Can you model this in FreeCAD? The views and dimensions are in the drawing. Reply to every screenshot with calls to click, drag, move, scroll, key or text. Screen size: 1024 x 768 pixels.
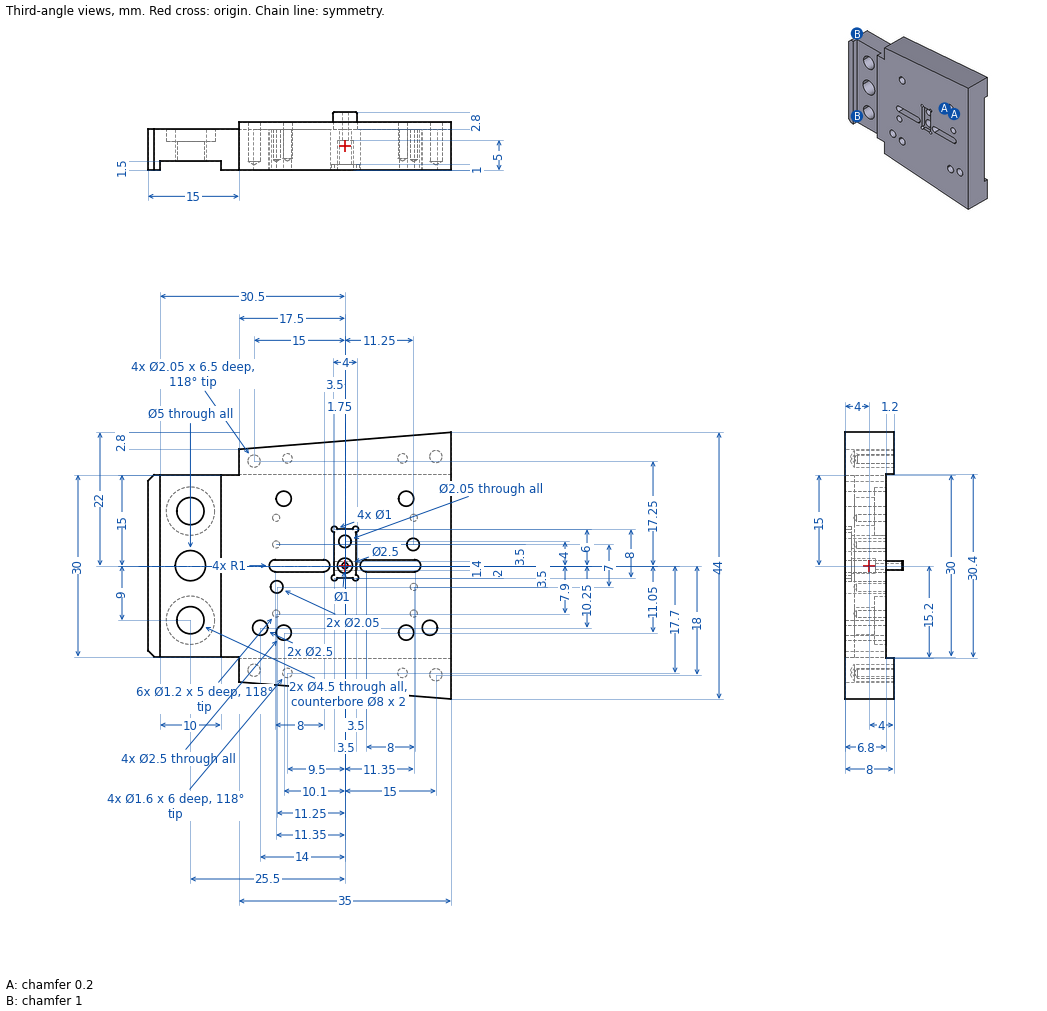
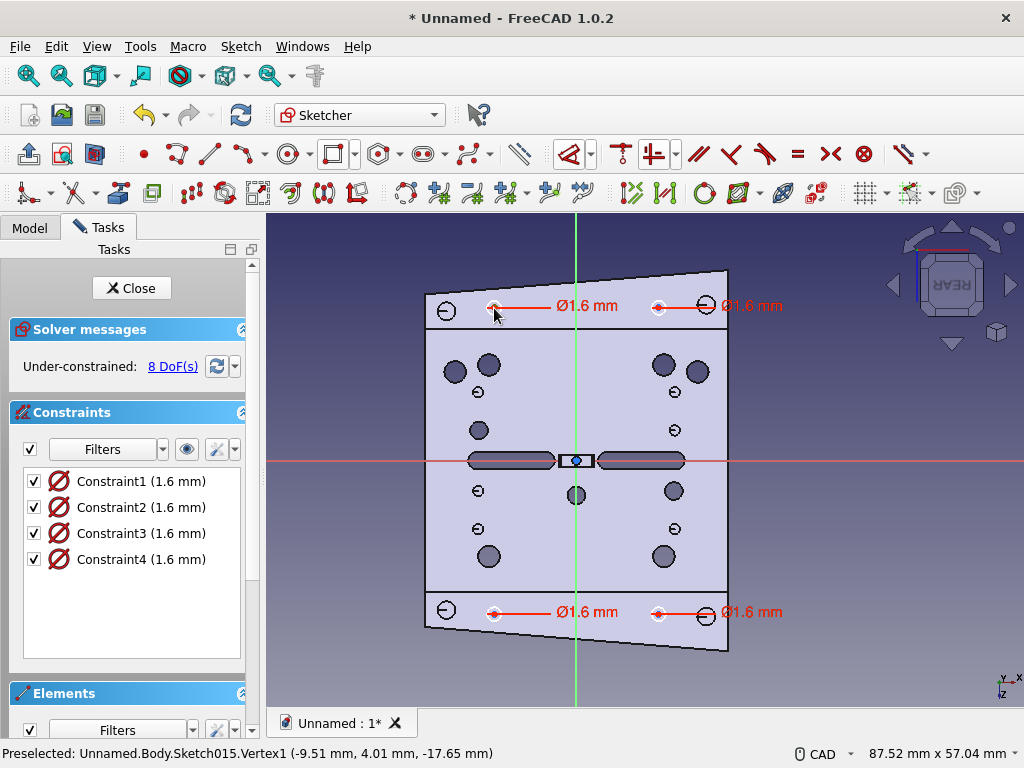
click(659, 308)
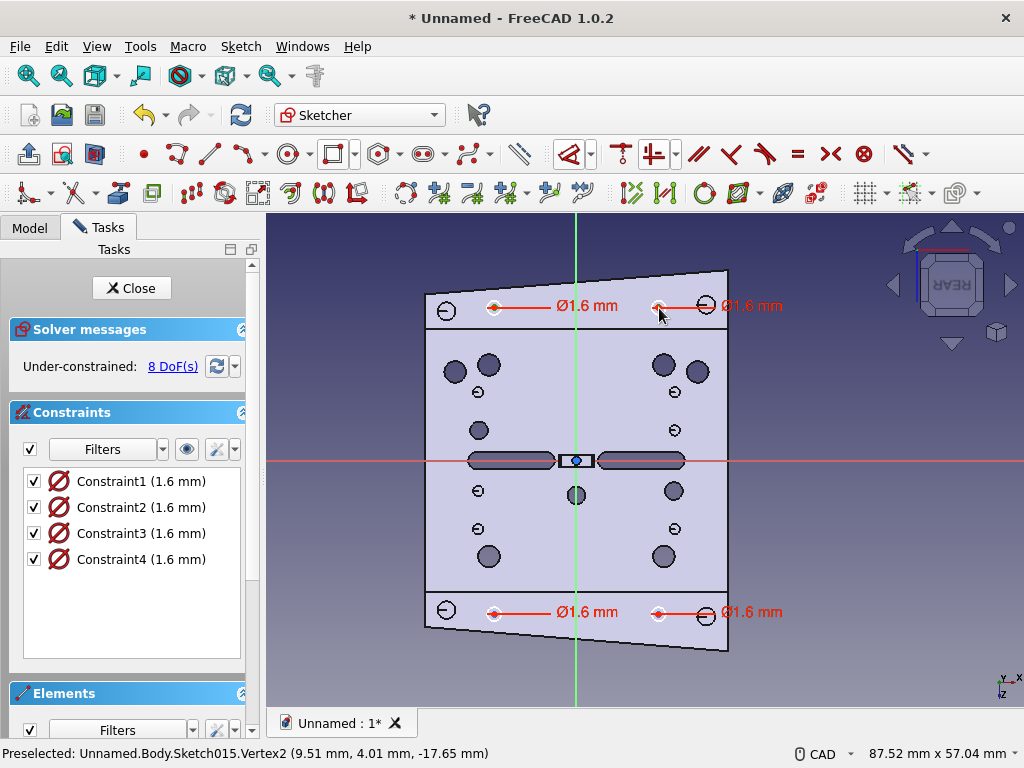
click(576, 648)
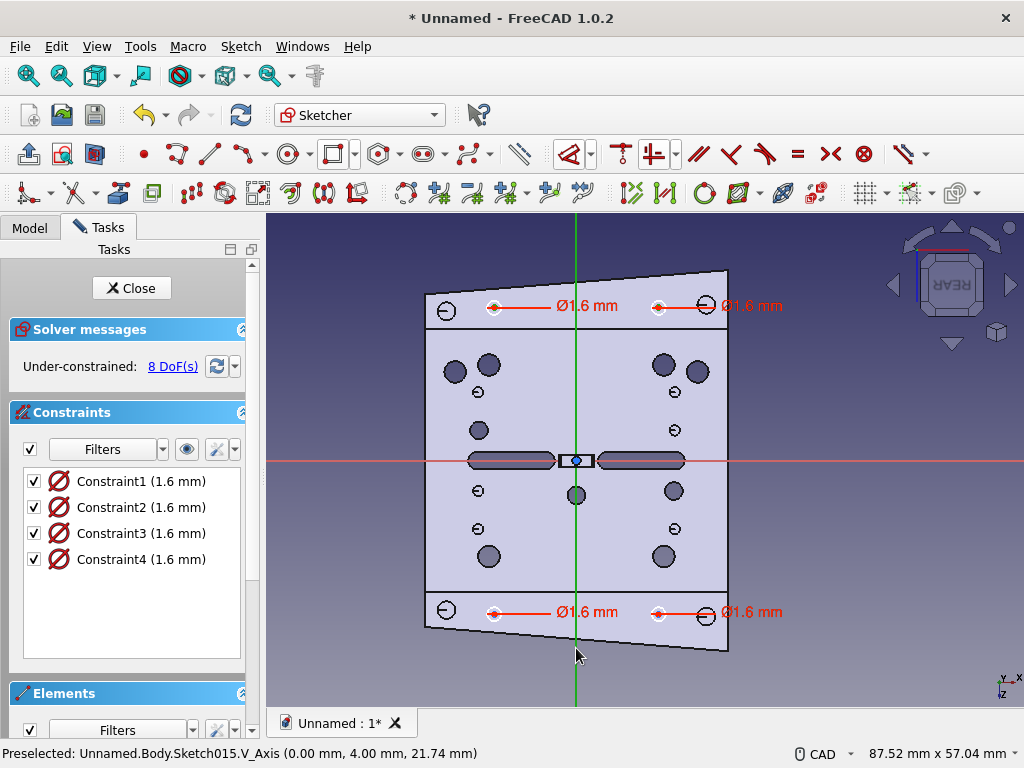
click(831, 154)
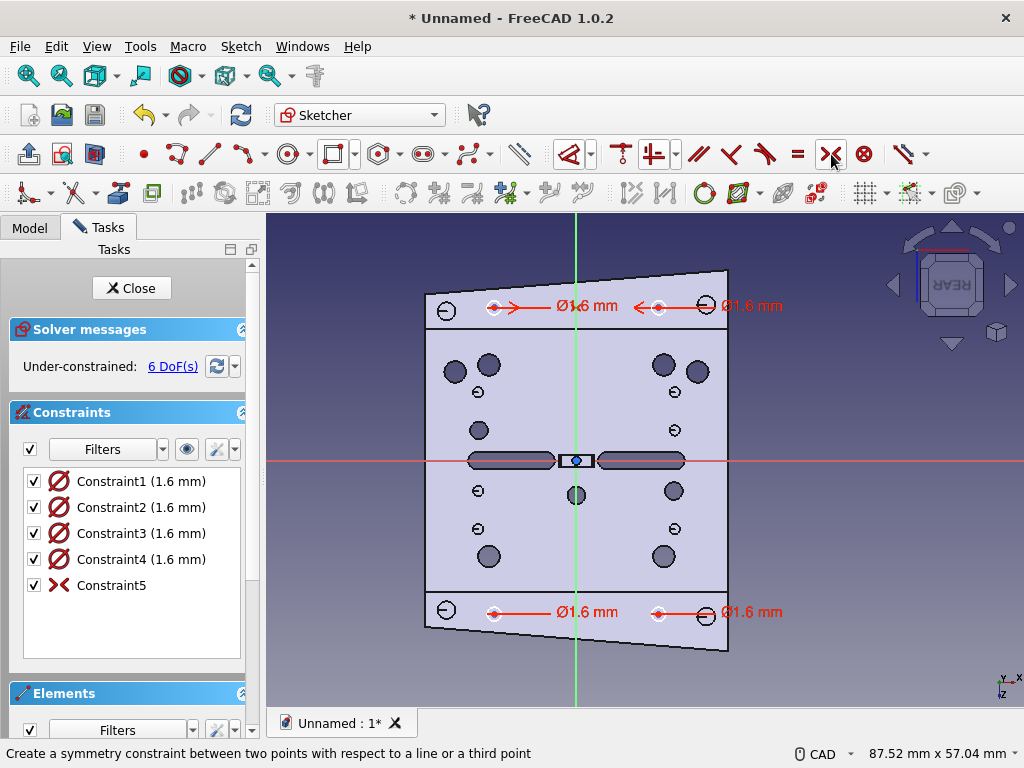
click(659, 308)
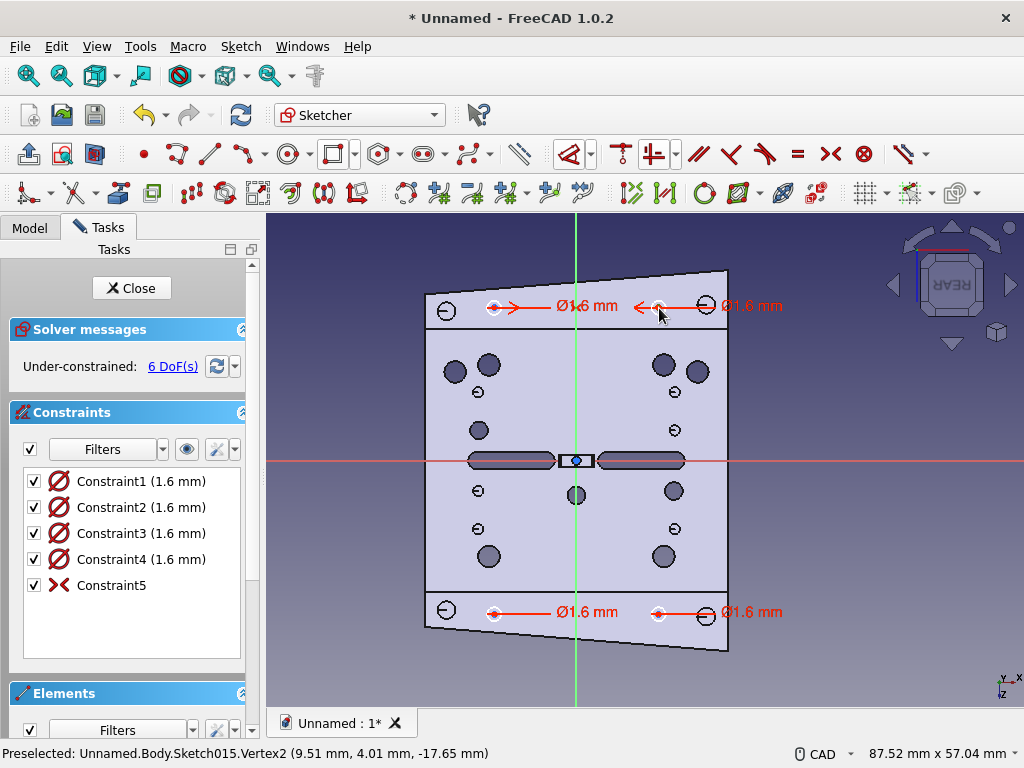
click(659, 614)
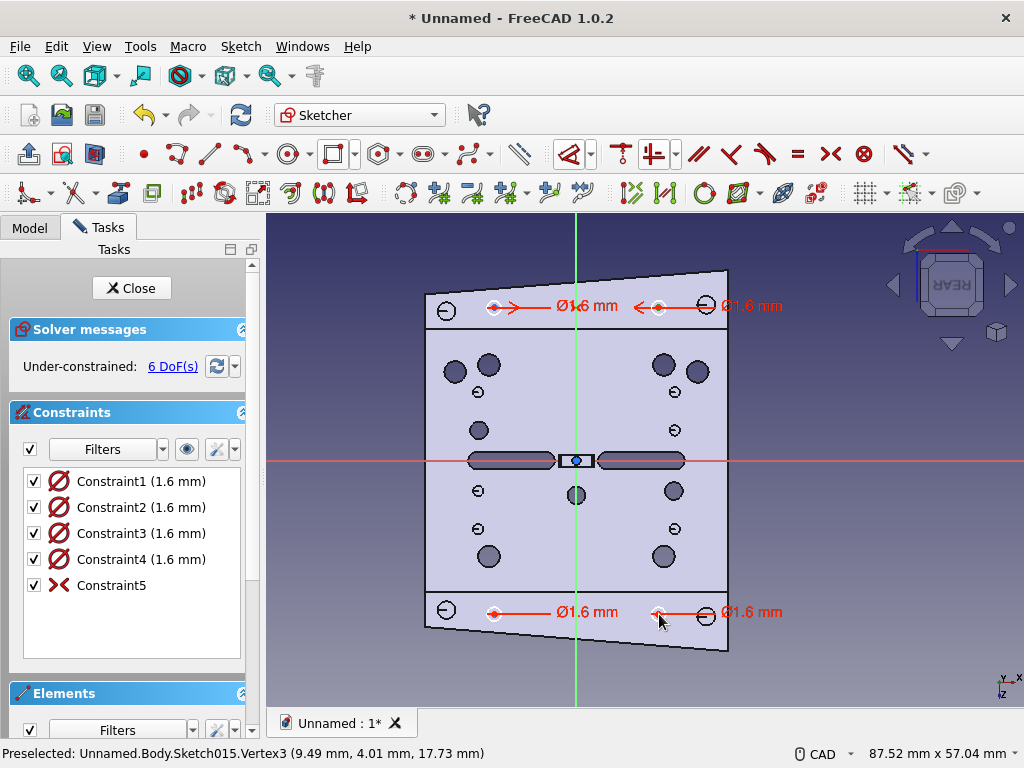
click(334, 461)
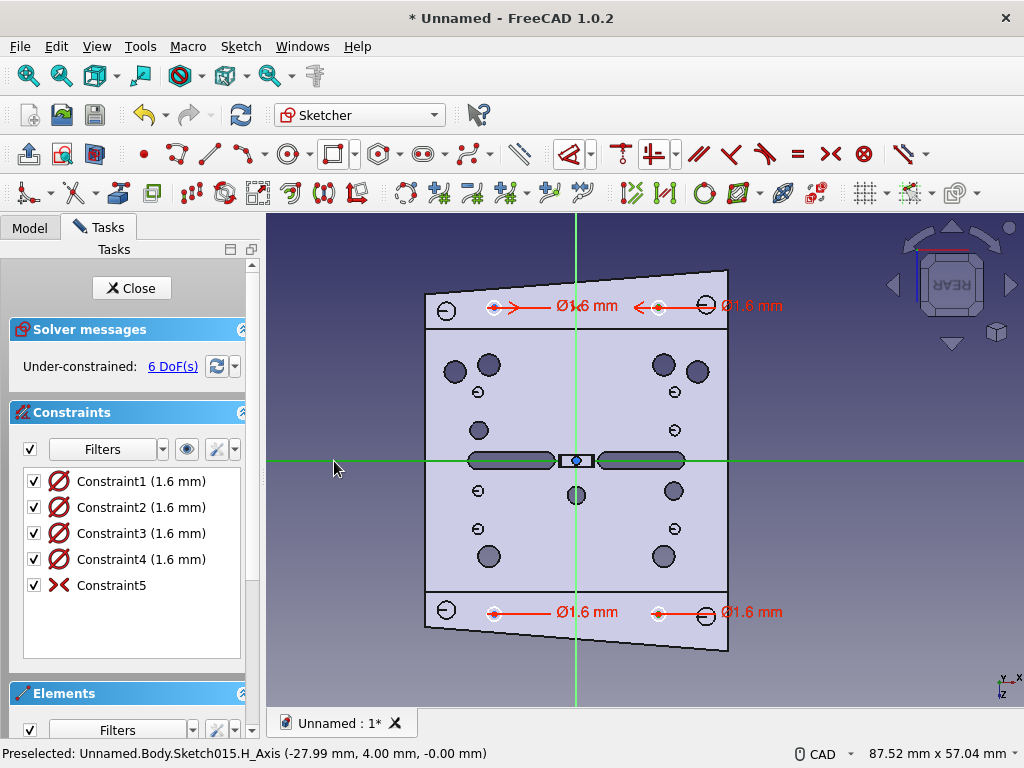
click(831, 154)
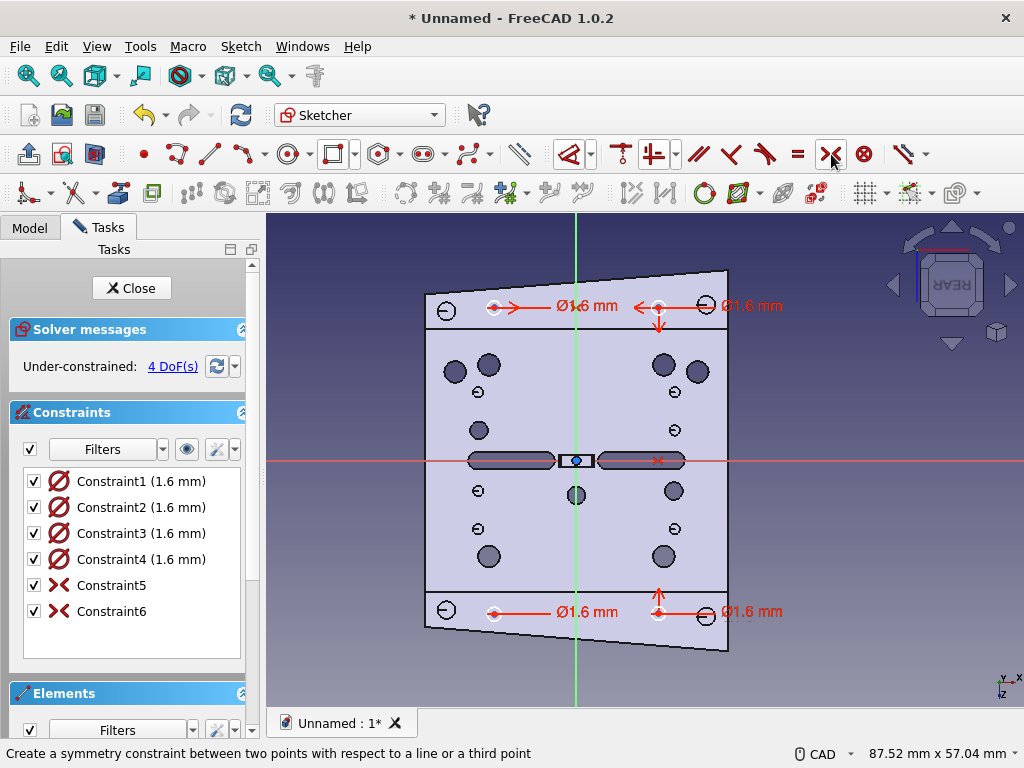
click(494, 308)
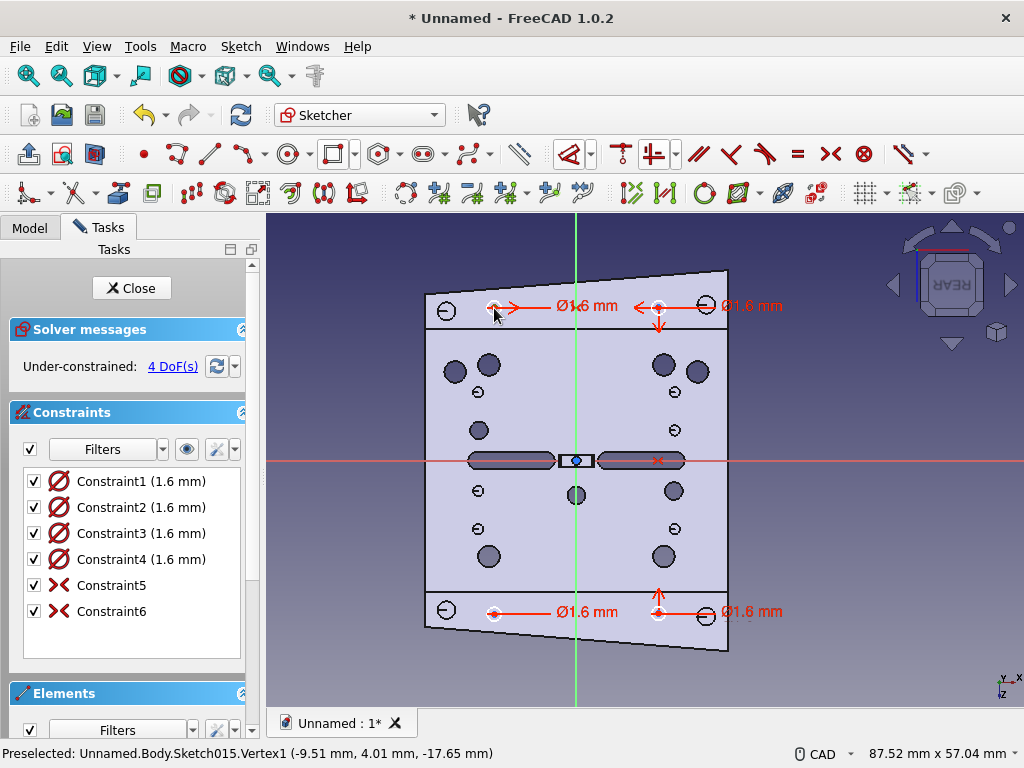
click(494, 614)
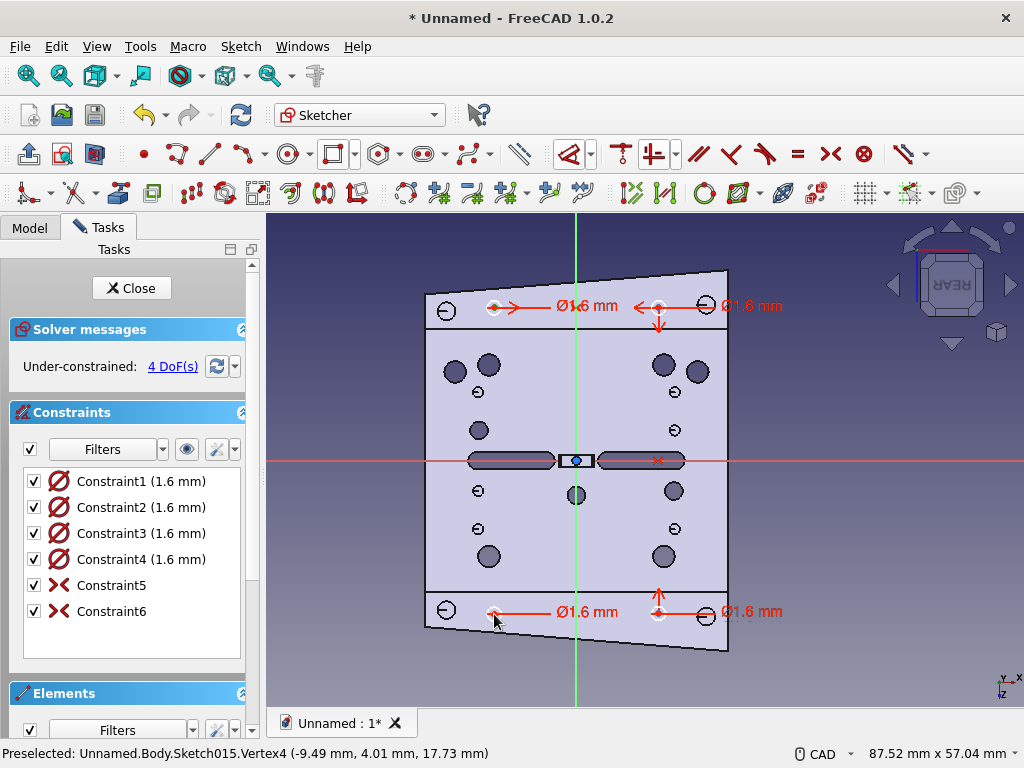
click(334, 461)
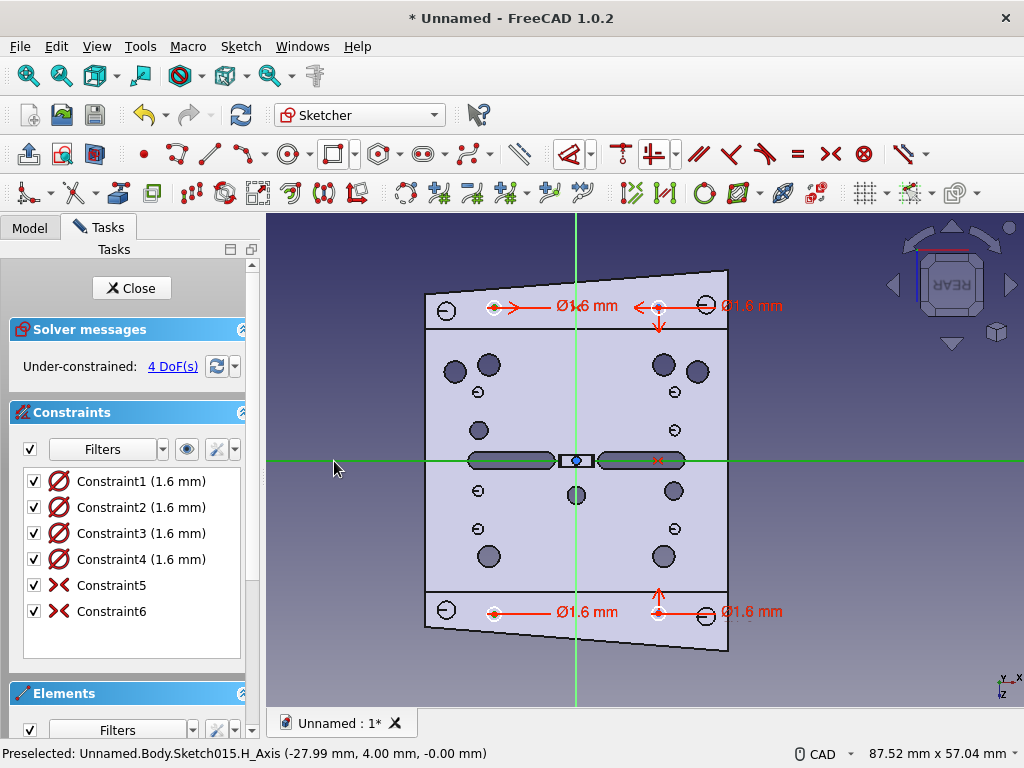
click(831, 154)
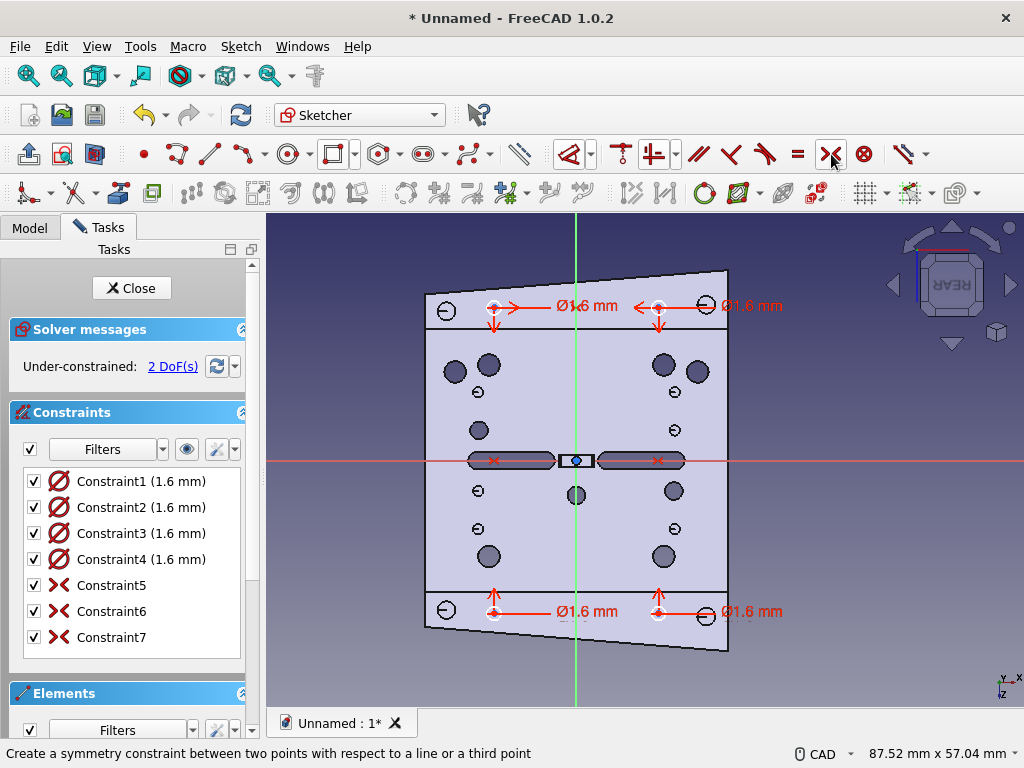
click(494, 308)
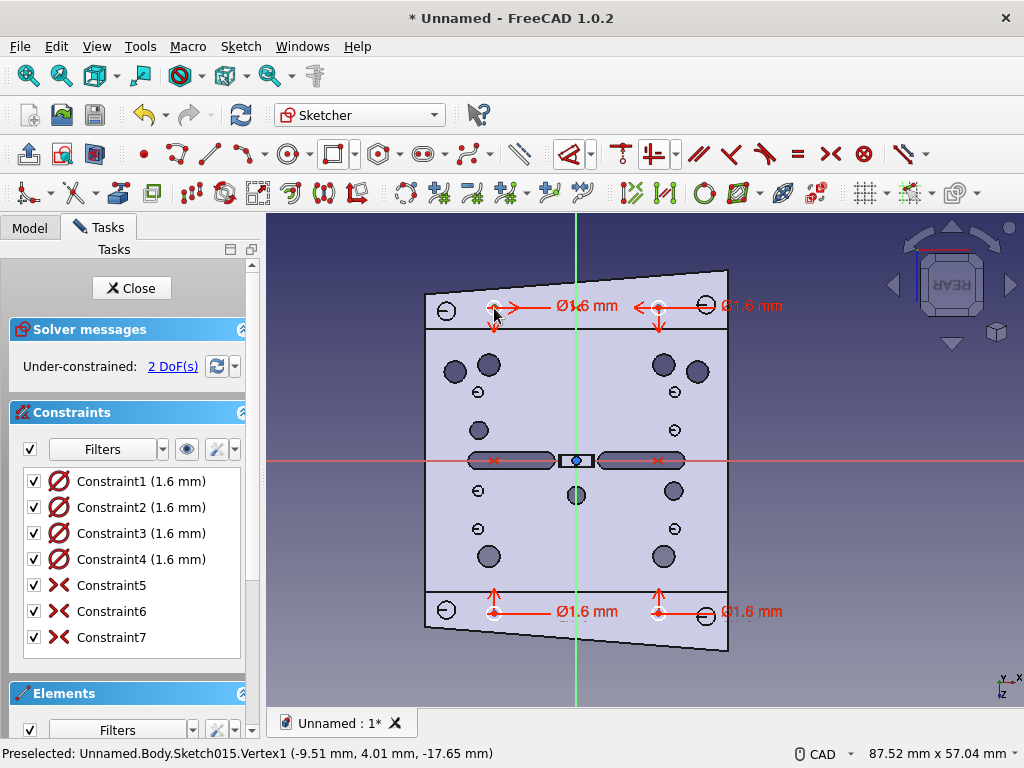
click(590, 154)